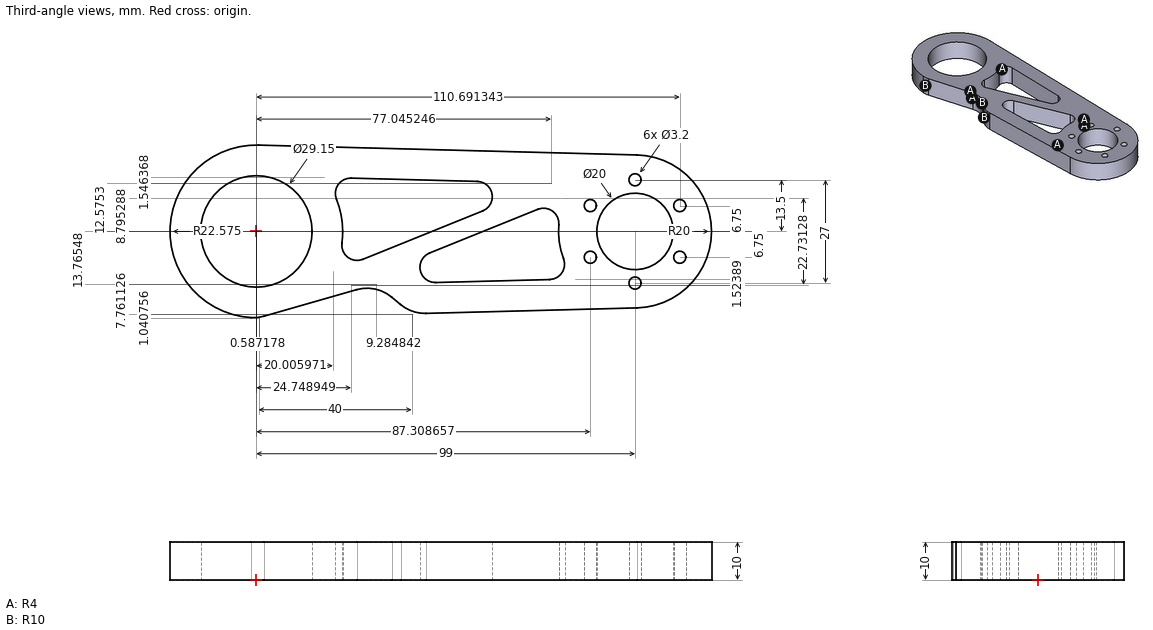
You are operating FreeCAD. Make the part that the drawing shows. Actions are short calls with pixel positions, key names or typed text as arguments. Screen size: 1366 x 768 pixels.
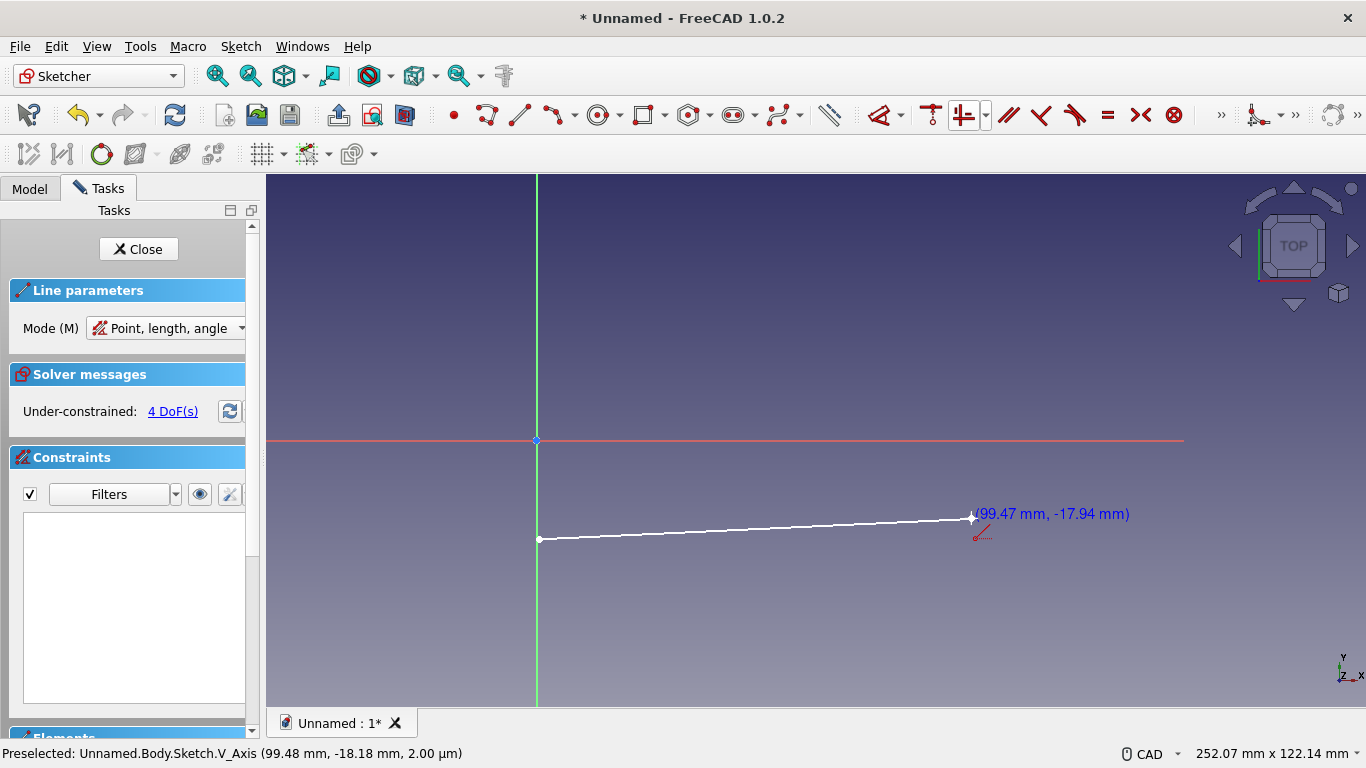
click(971, 353)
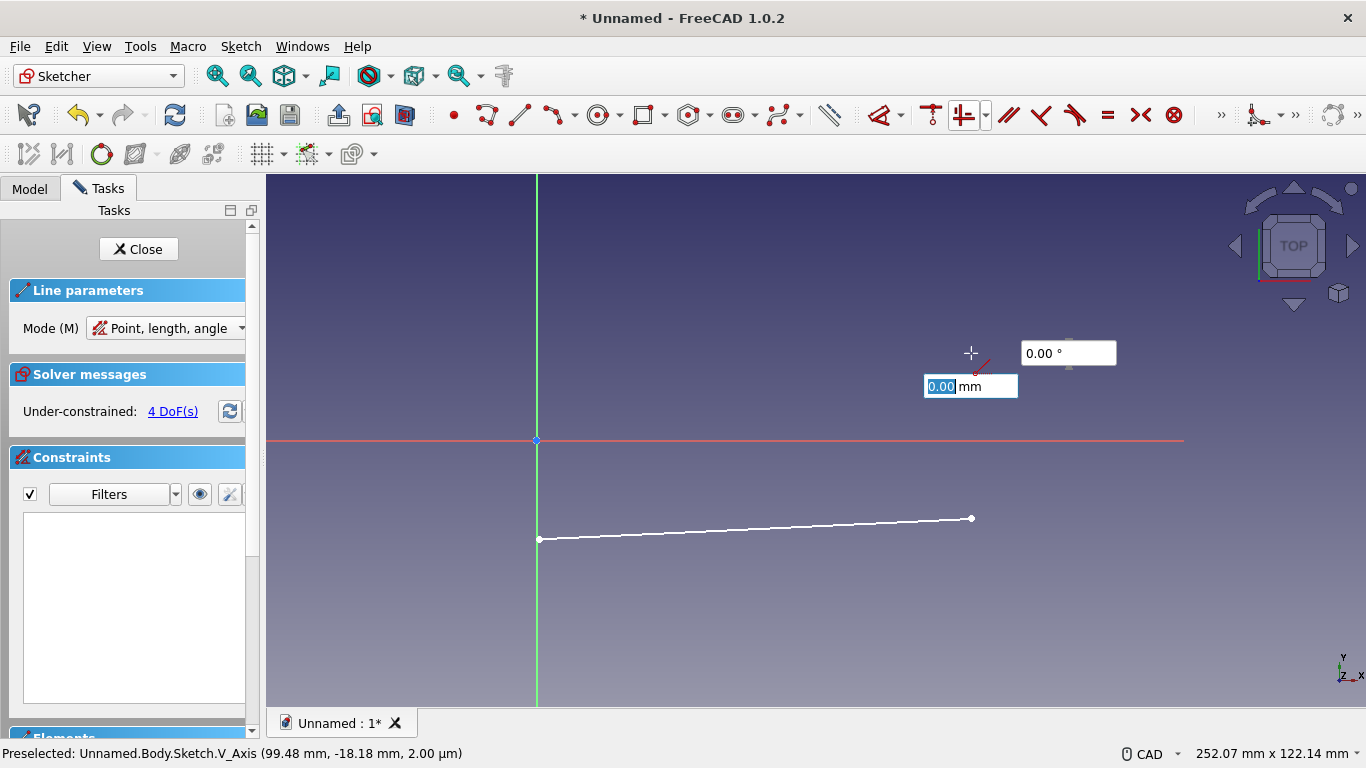
scroll(539, 342, up, 10)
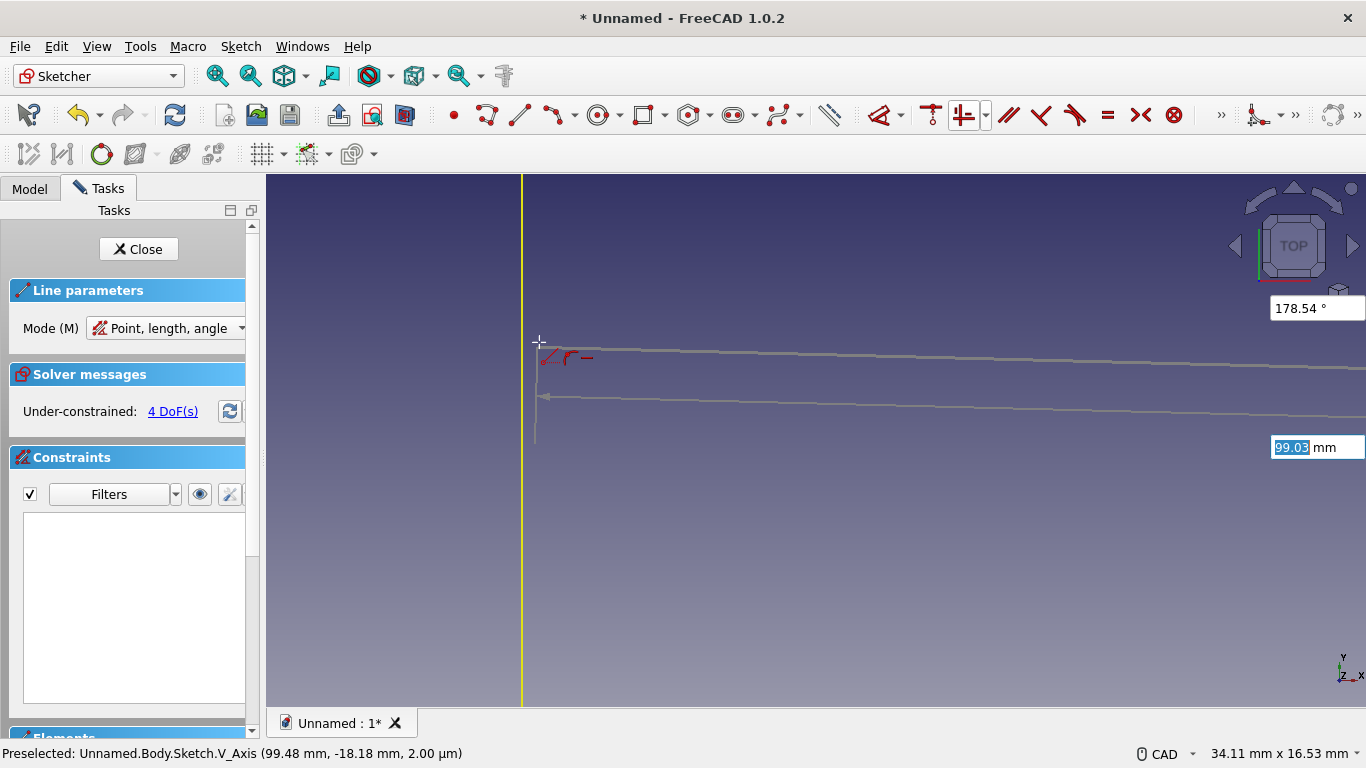
click(541, 276)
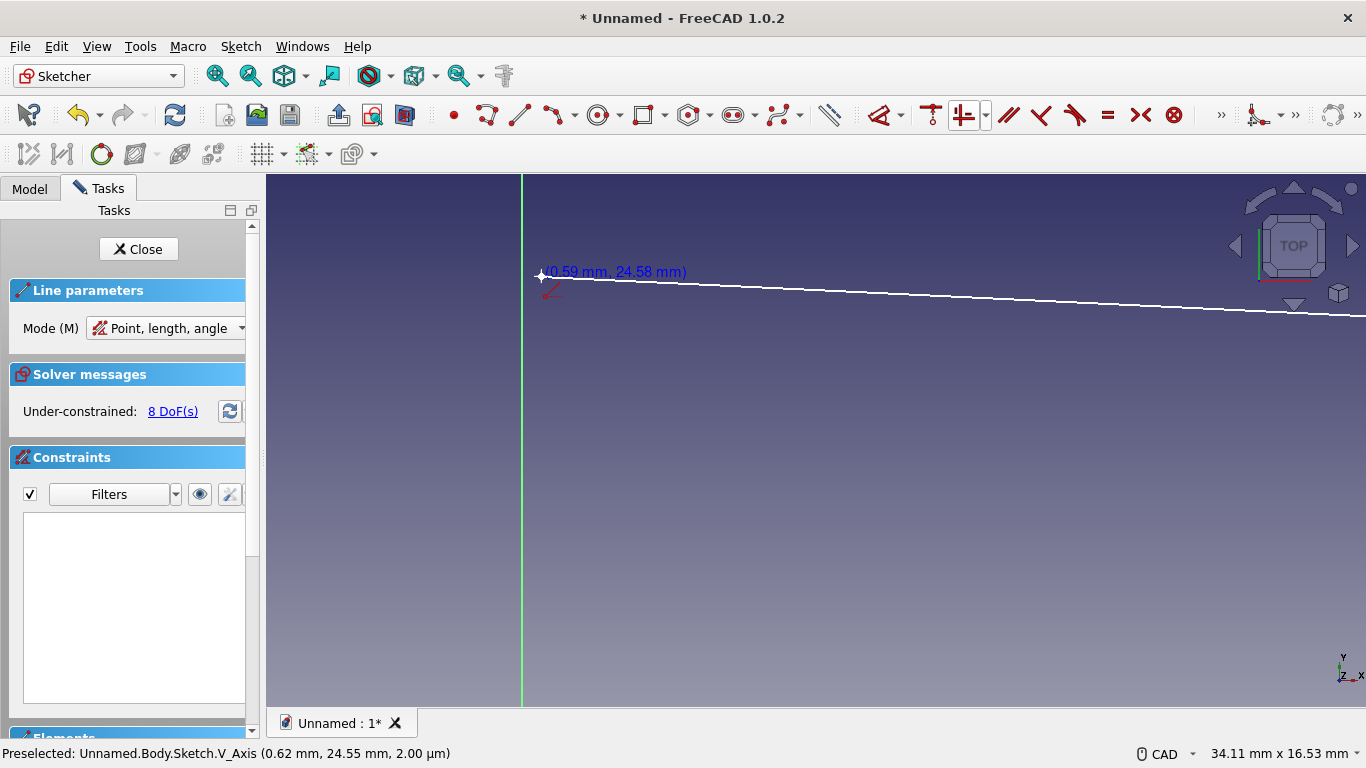
key(g)
key(3)
key(a)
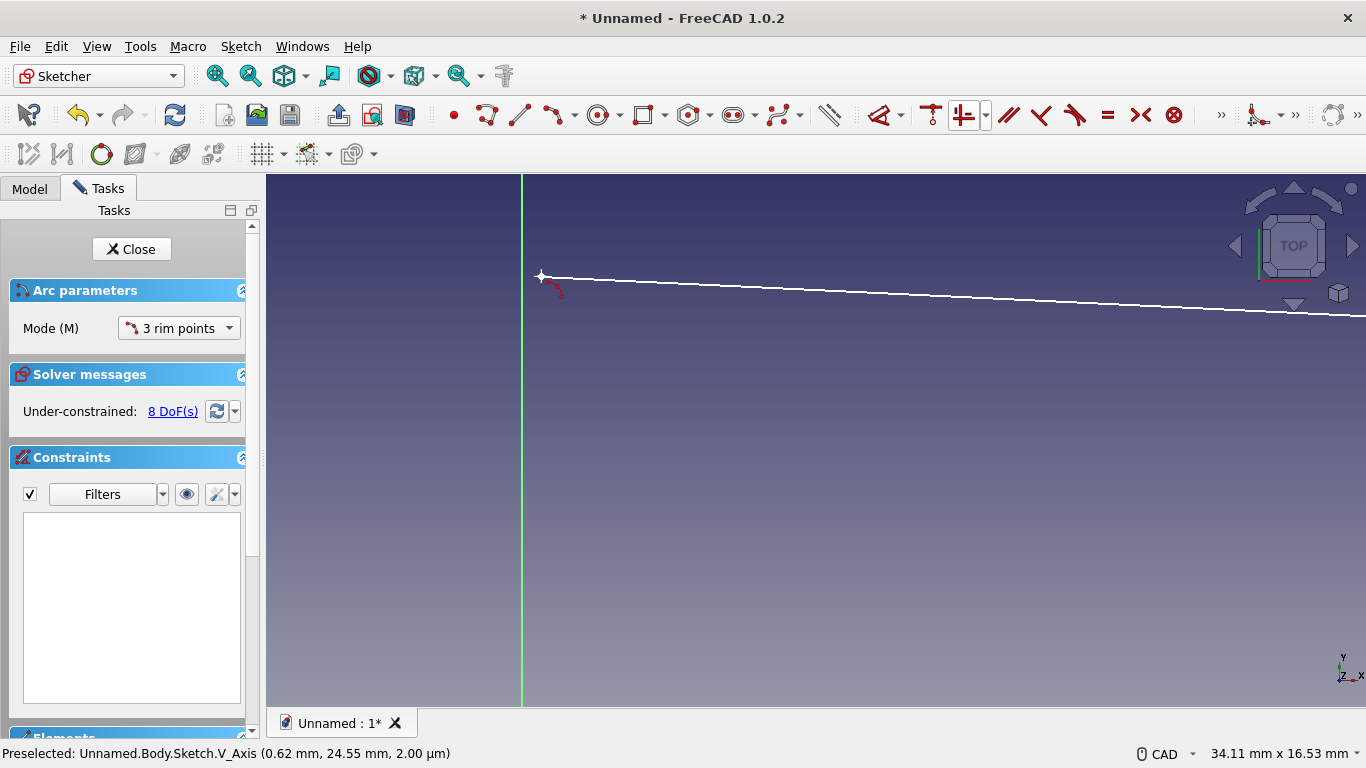
scroll(539, 342, down, 10)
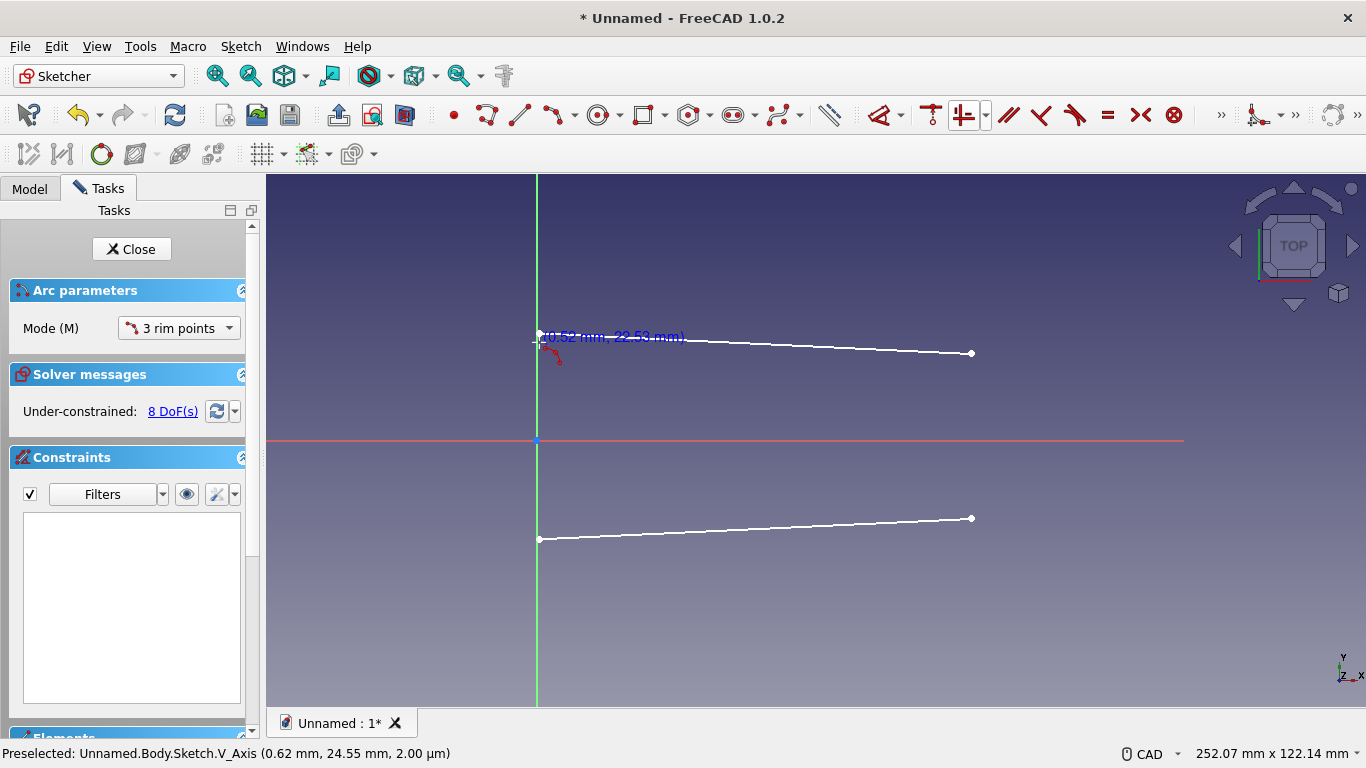
click(971, 519)
click(971, 354)
click(1052, 467)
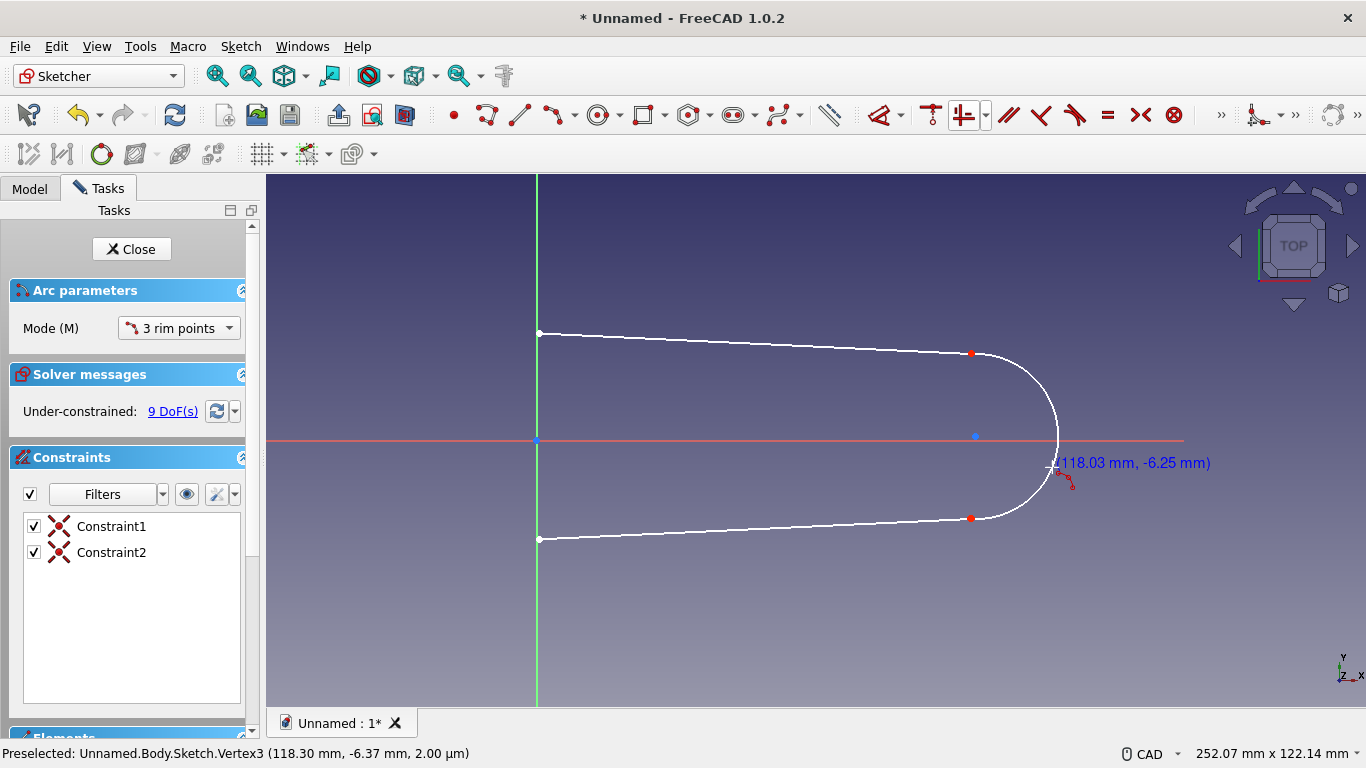
scroll(539, 342, up, 10)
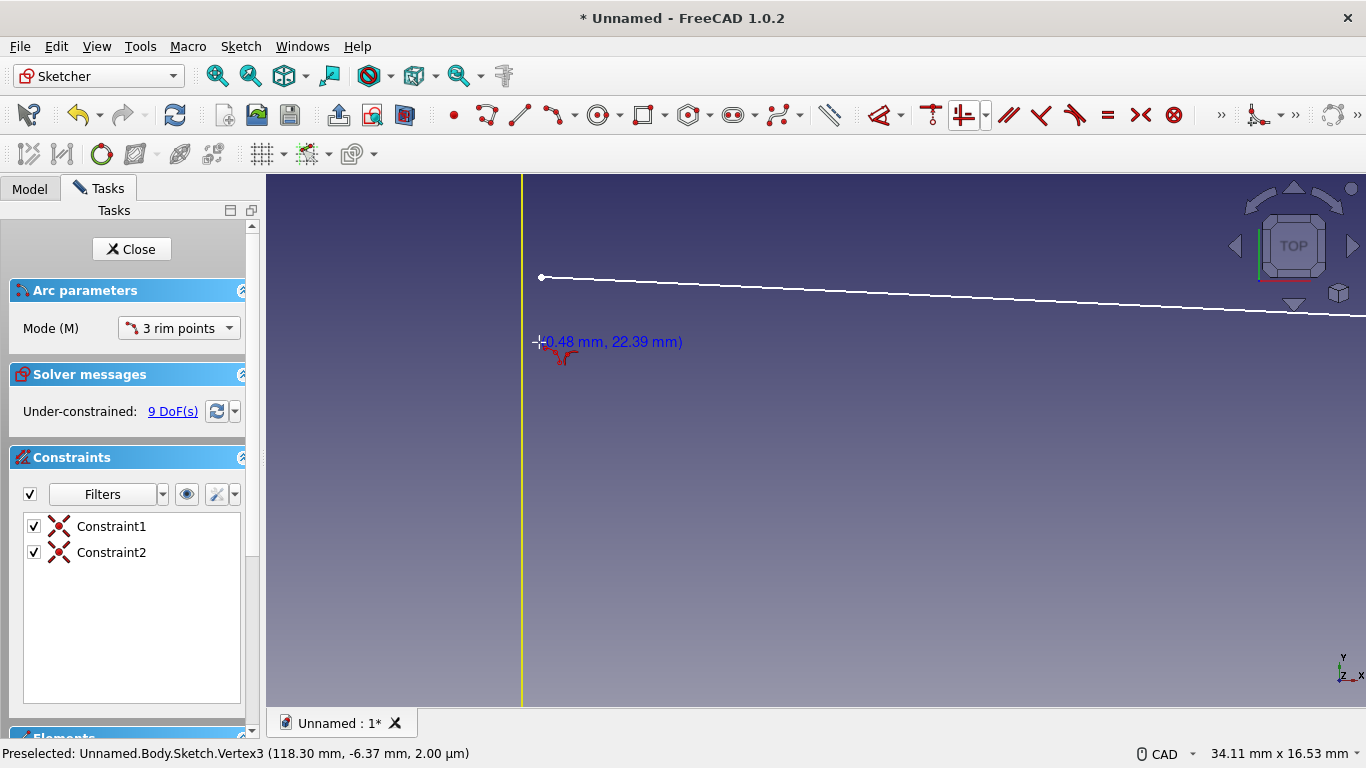
click(541, 277)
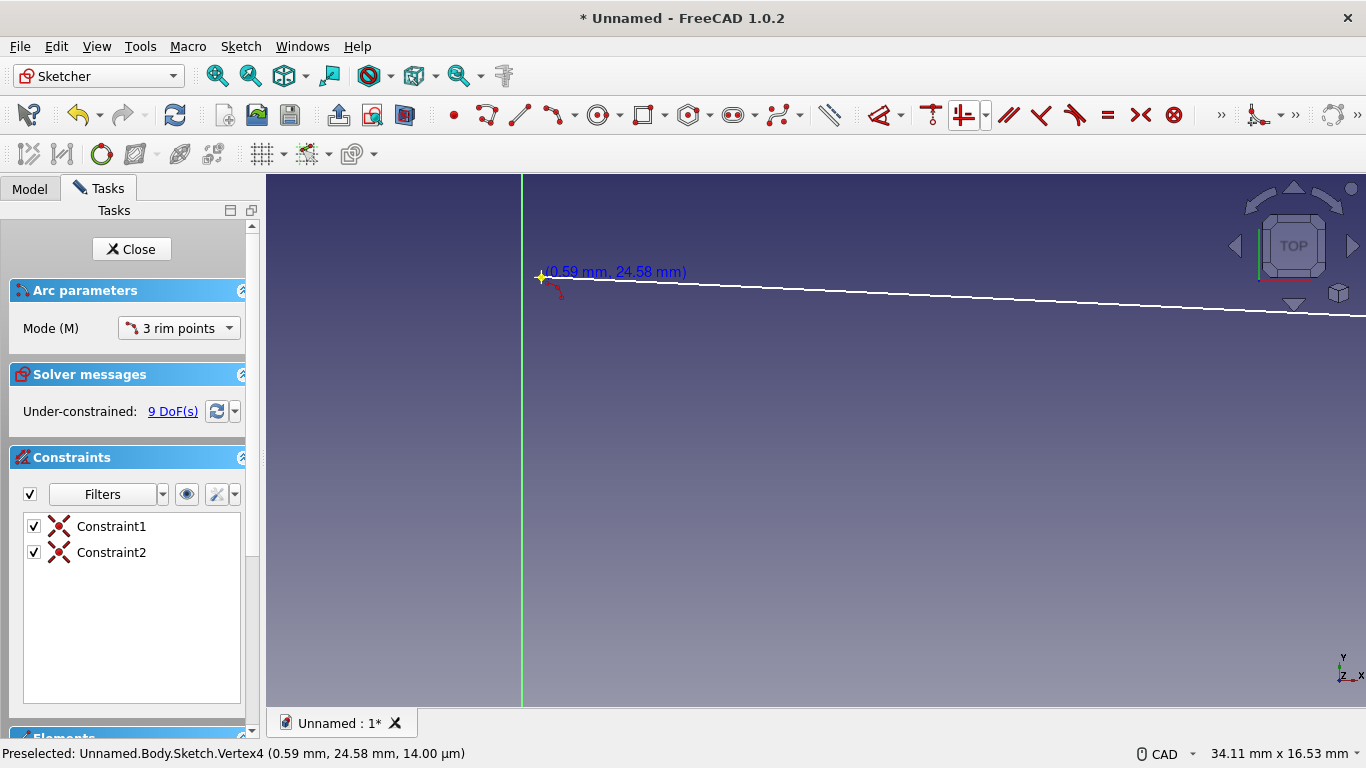
scroll(539, 342, down, 10)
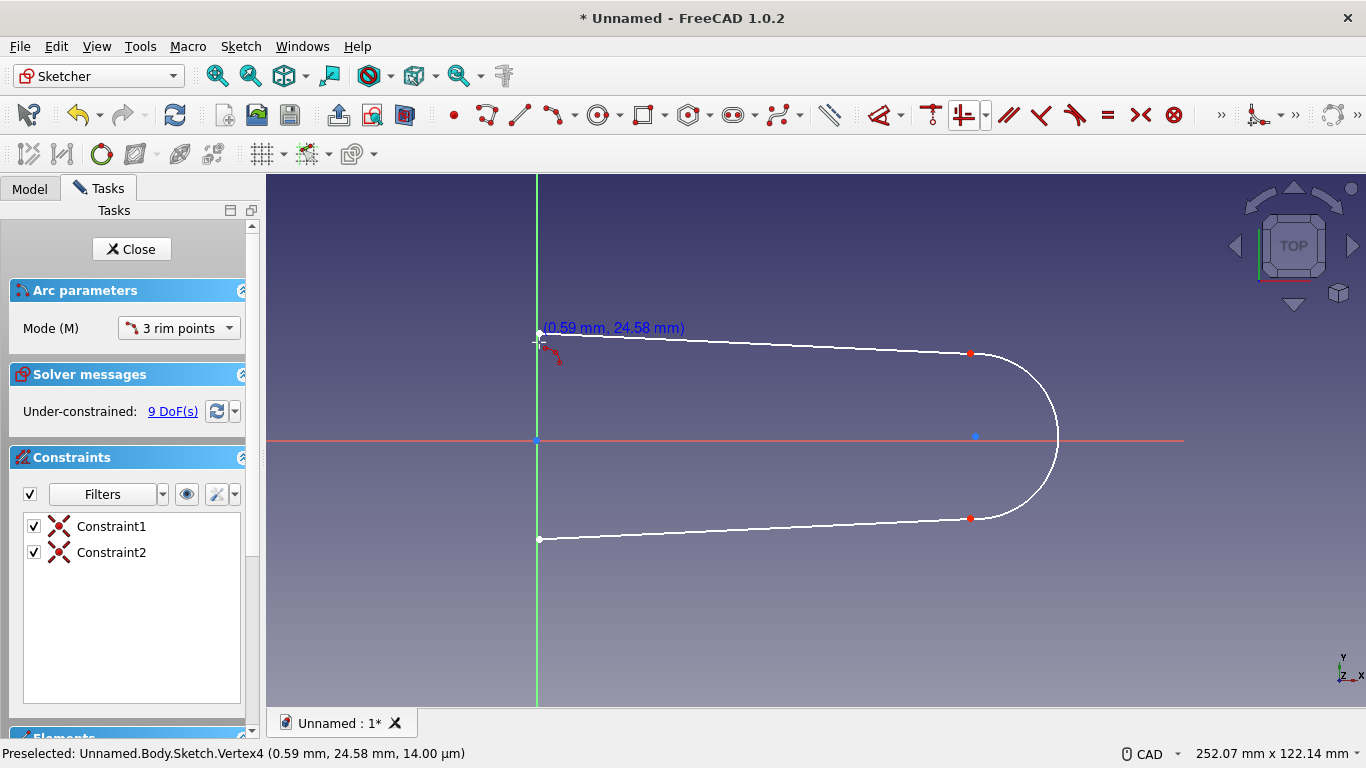
scroll(539, 539, up, 10)